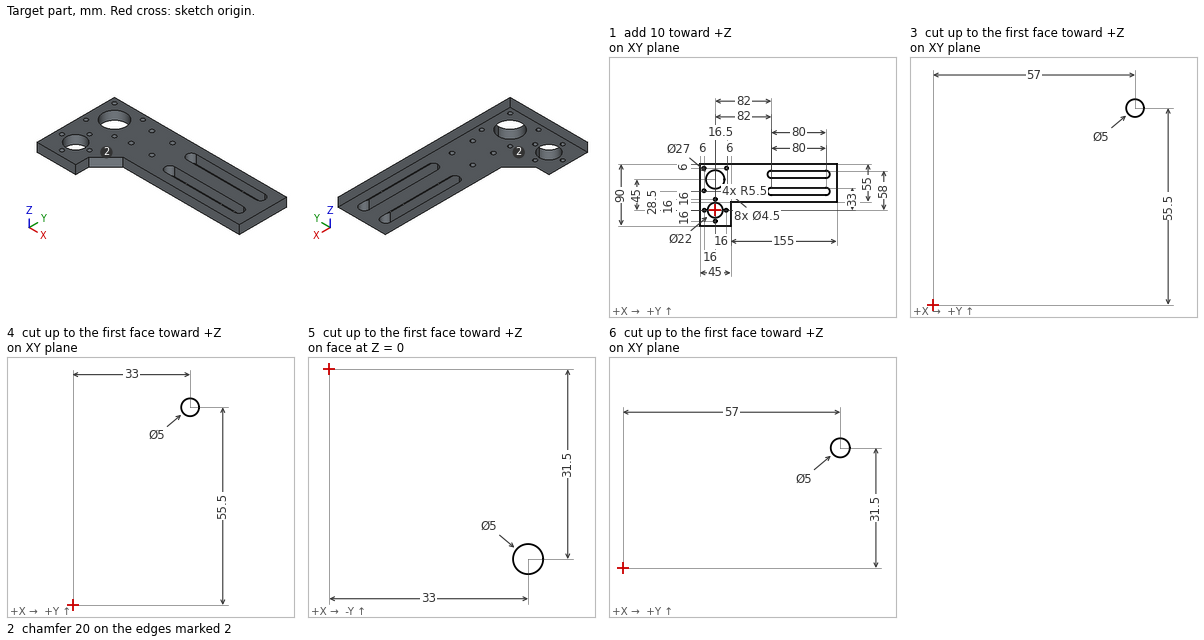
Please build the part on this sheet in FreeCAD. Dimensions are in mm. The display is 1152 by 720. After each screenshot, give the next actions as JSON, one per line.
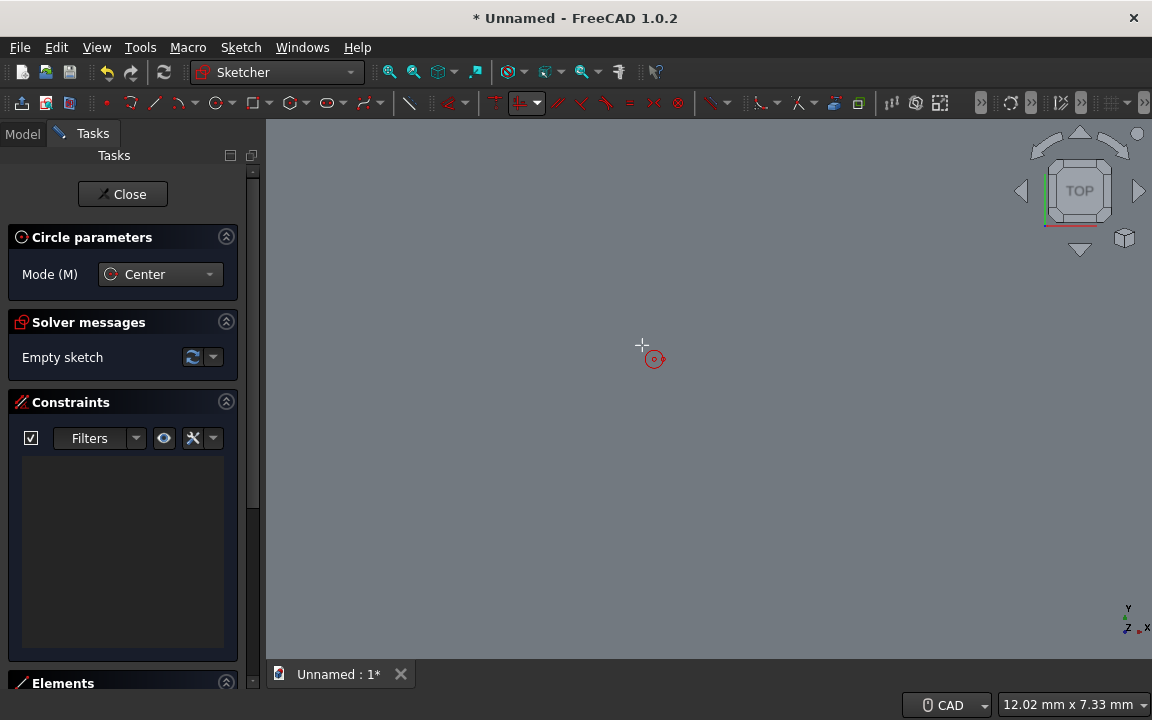
{"action": "left_click", "coordinate": [640, 389]}
{"action": "mouse_move", "coordinate": [771, 258]}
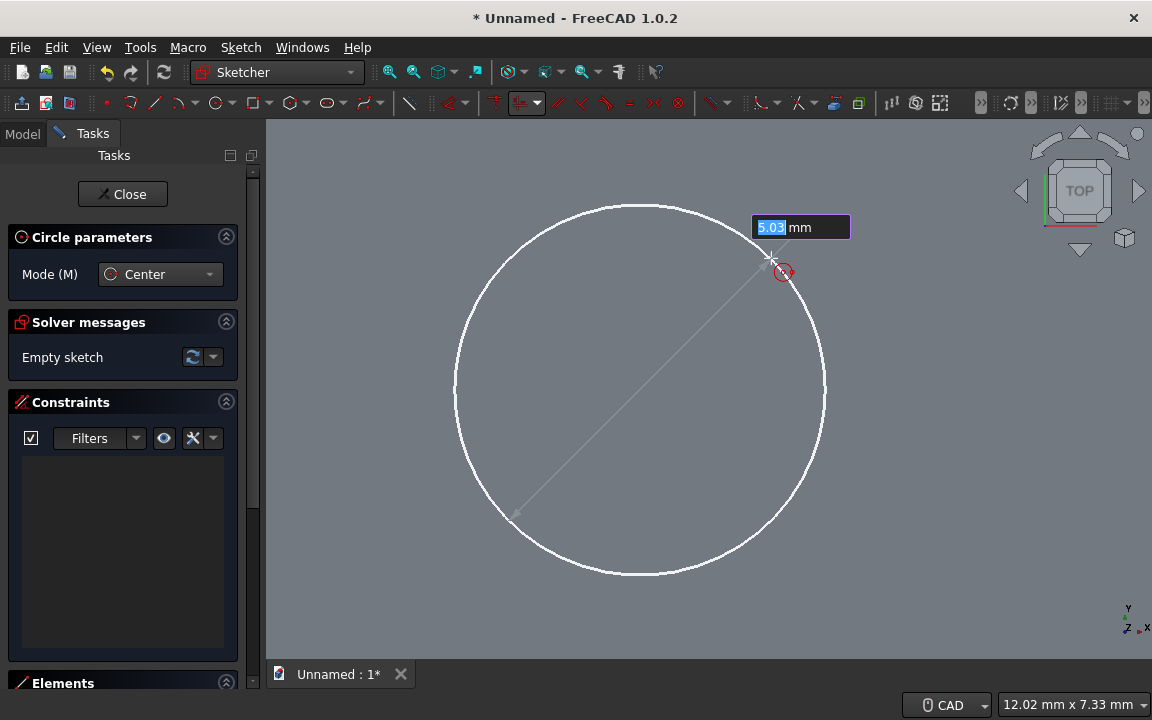
{"action": "type", "text": "5"}
{"action": "key", "text": "Return"}
{"action": "key", "text": "Escape"}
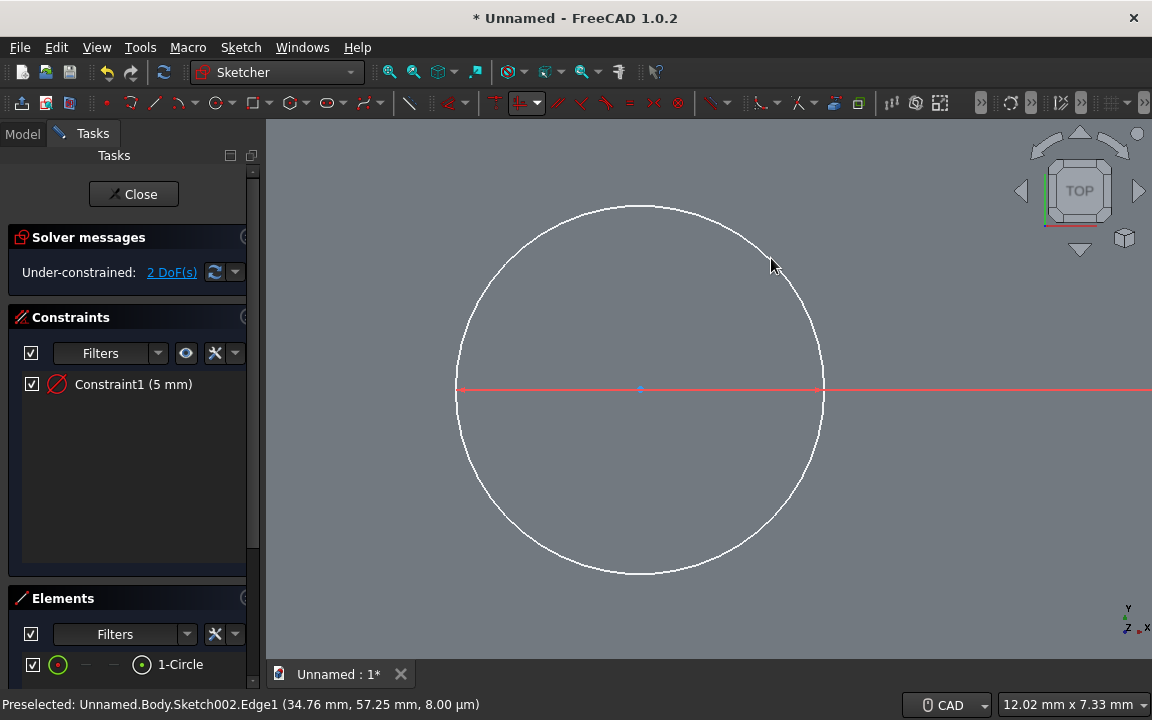
{"action": "key", "text": "d"}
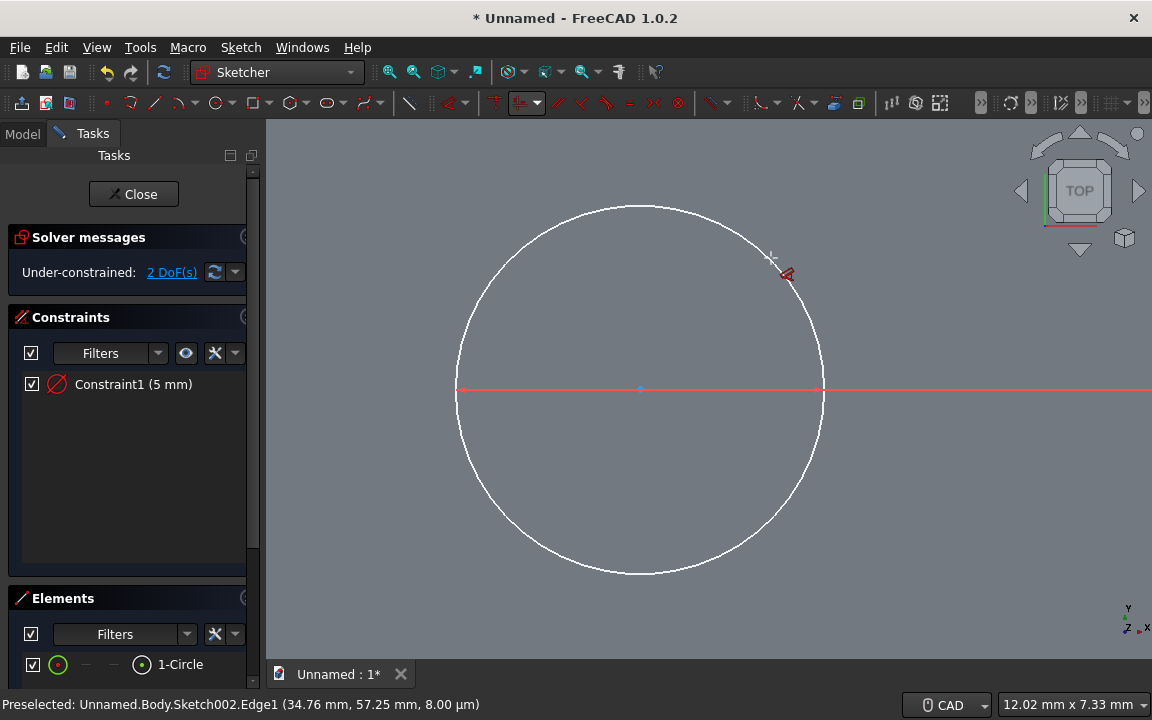
{"action": "left_click", "coordinate": [640, 390]}
{"action": "left_click", "coordinate": [387, 356]}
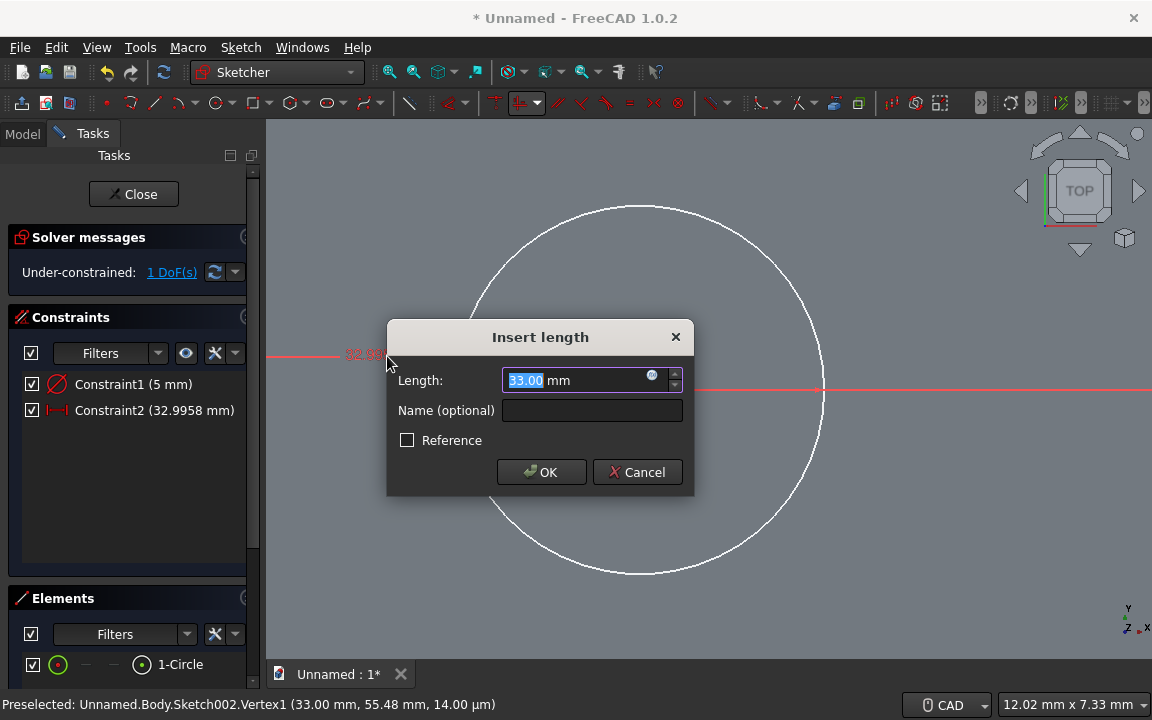
{"action": "type", "text": "33"}
{"action": "key", "text": "Return"}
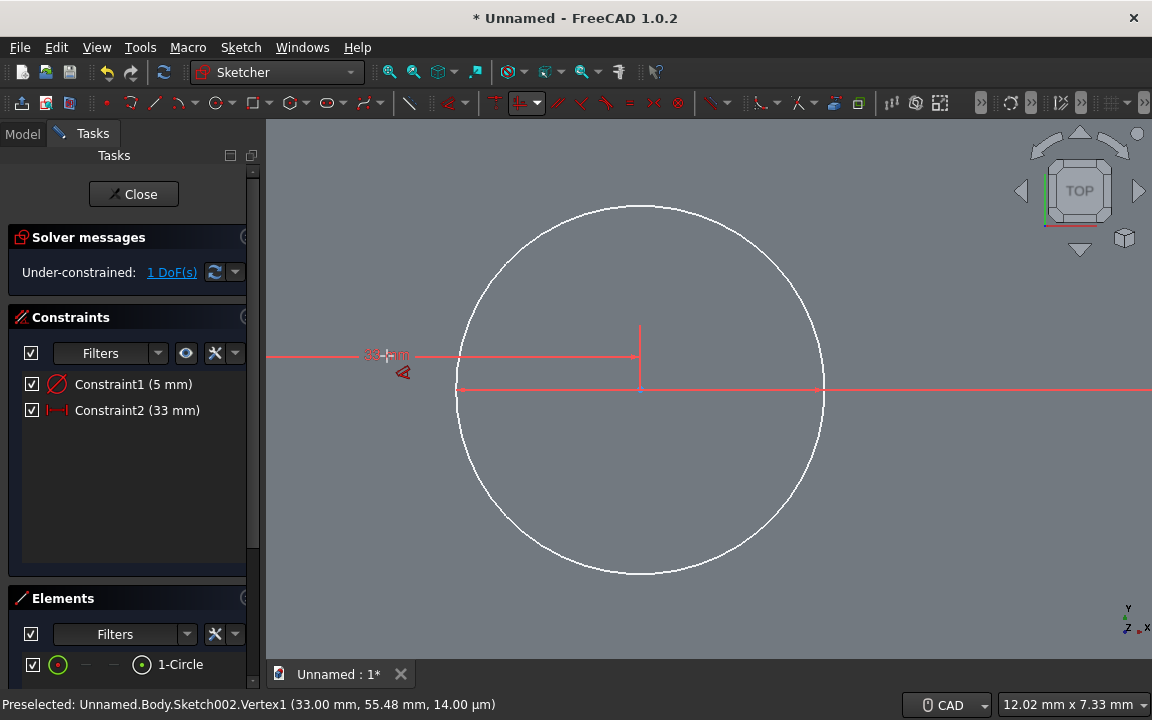
{"action": "left_click", "coordinate": [640, 390]}
{"action": "left_click", "coordinate": [674, 511]}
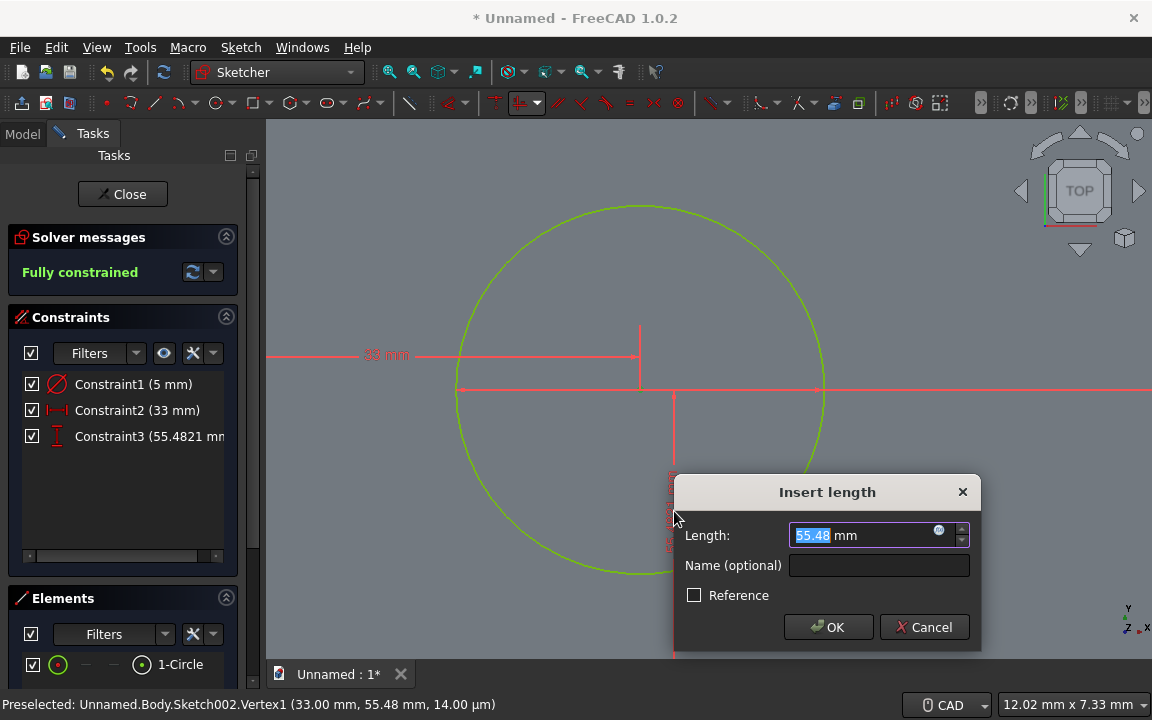
{"action": "type", "text": "55.5"}
{"action": "key", "text": "Return"}
{"action": "key", "text": "Escape"}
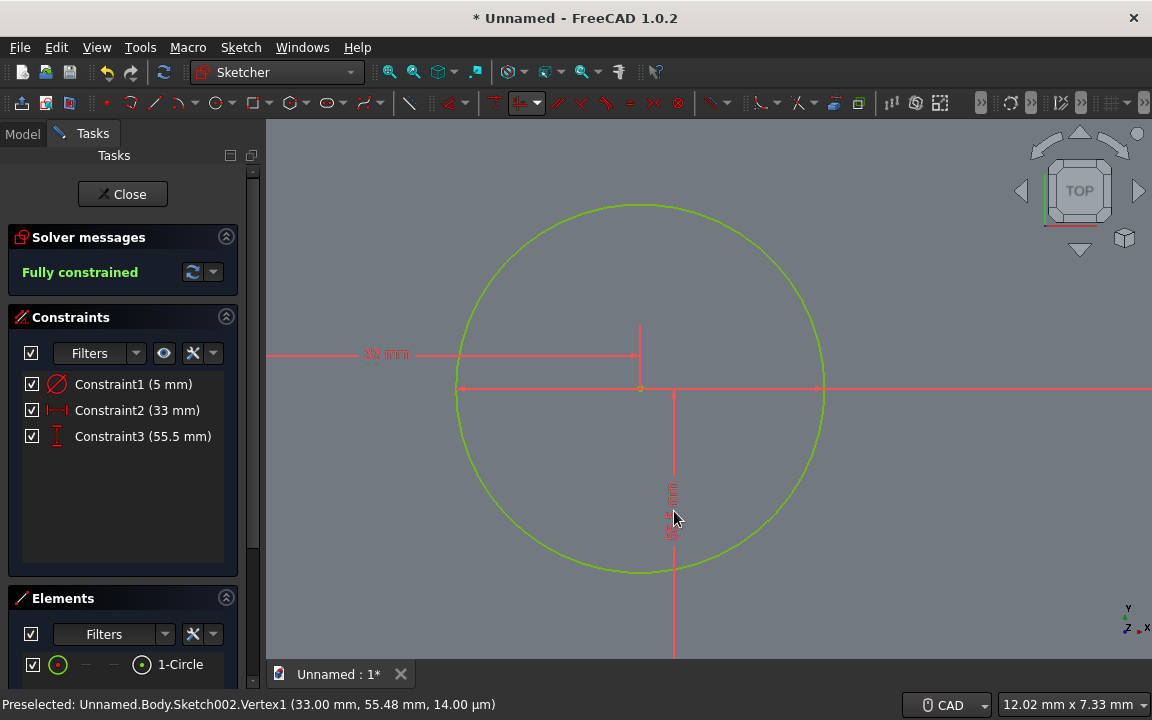
{"action": "left_click", "coordinate": [123, 194]}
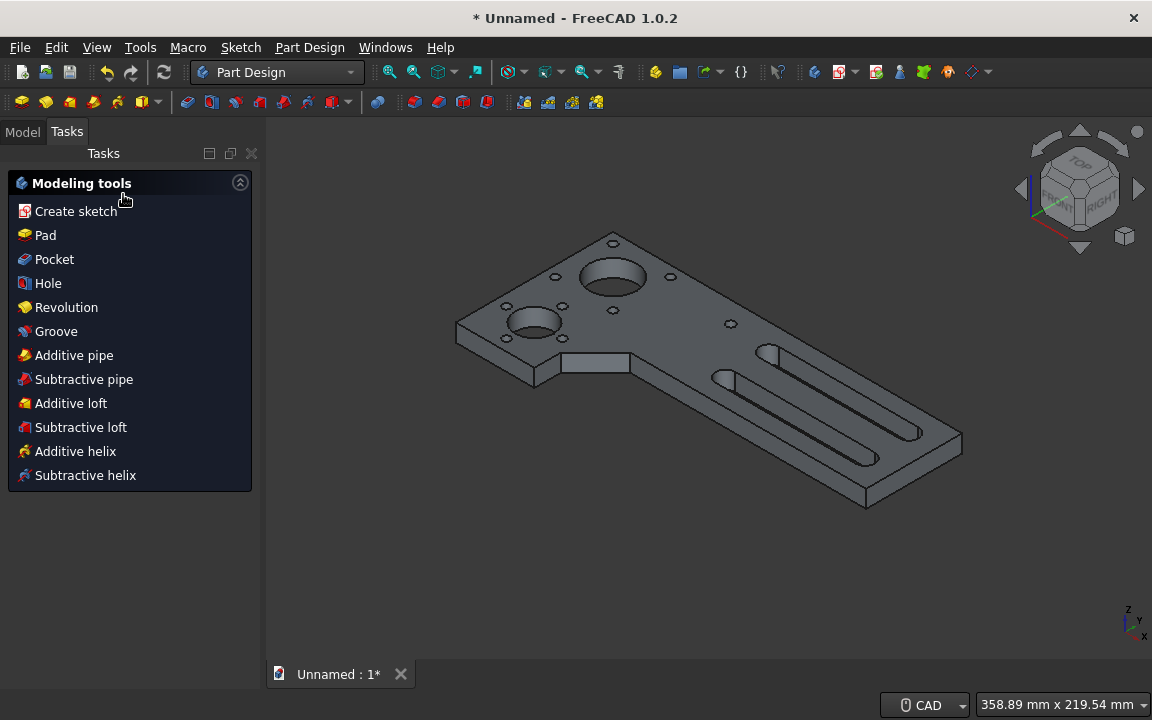
{"action": "left_click", "coordinate": [188, 102]}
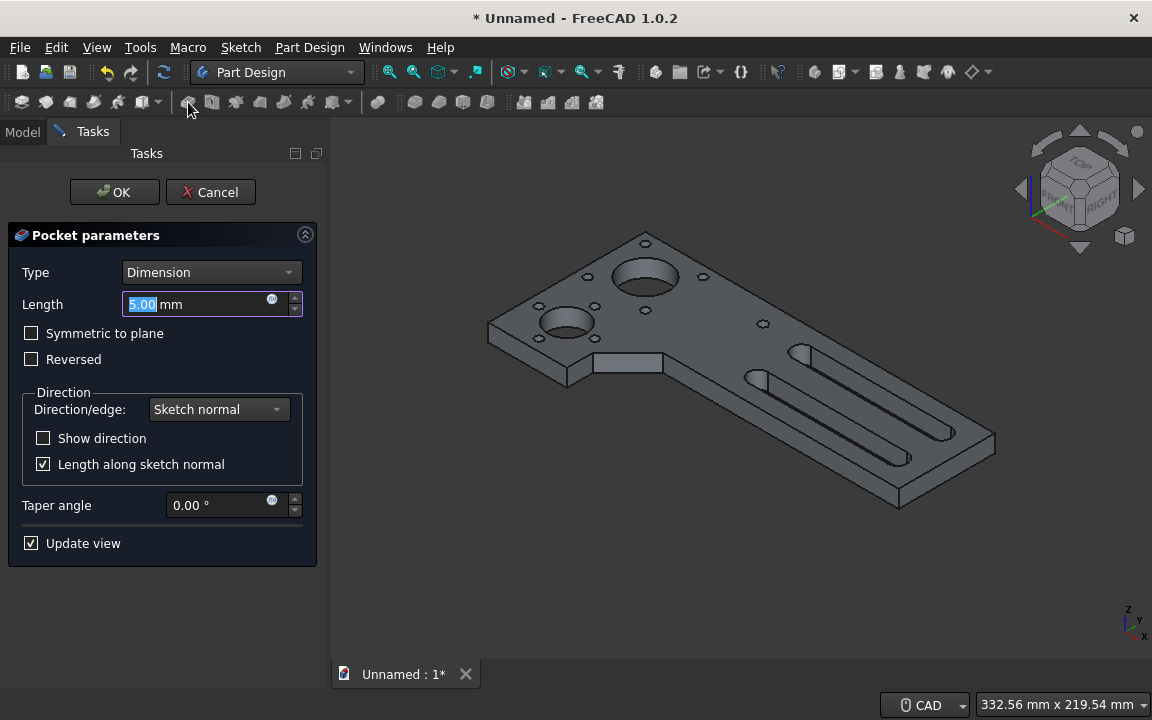
{"action": "left_click", "coordinate": [212, 272]}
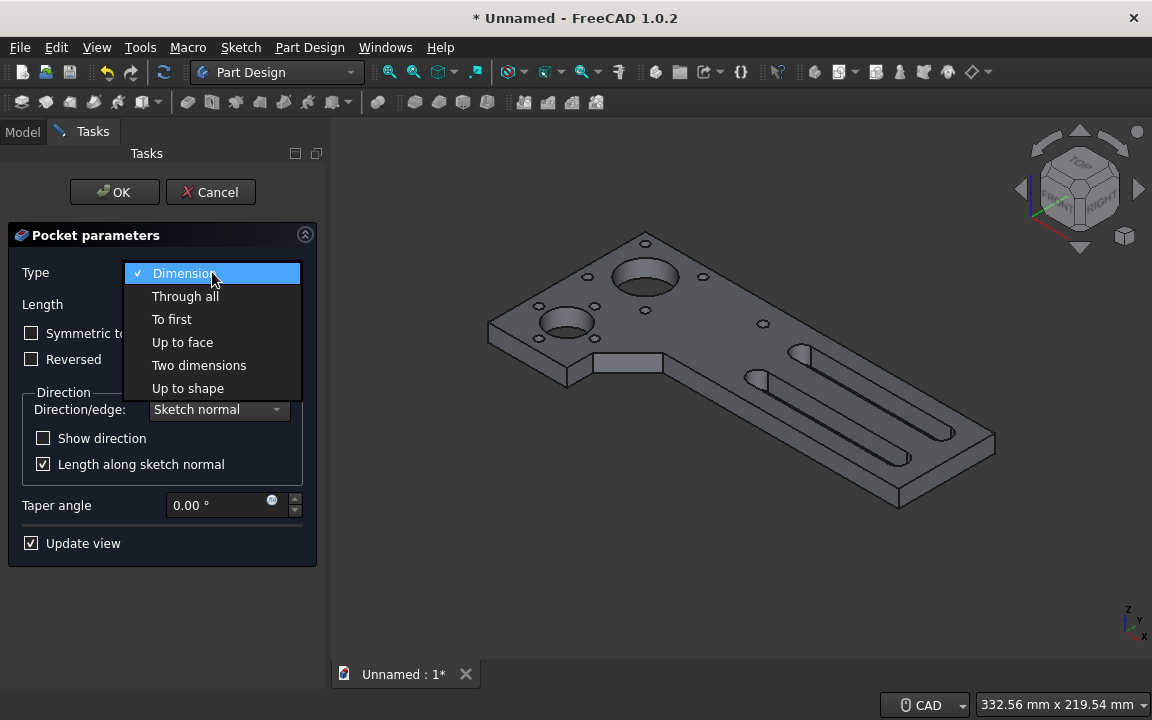
{"action": "left_click", "coordinate": [212, 320]}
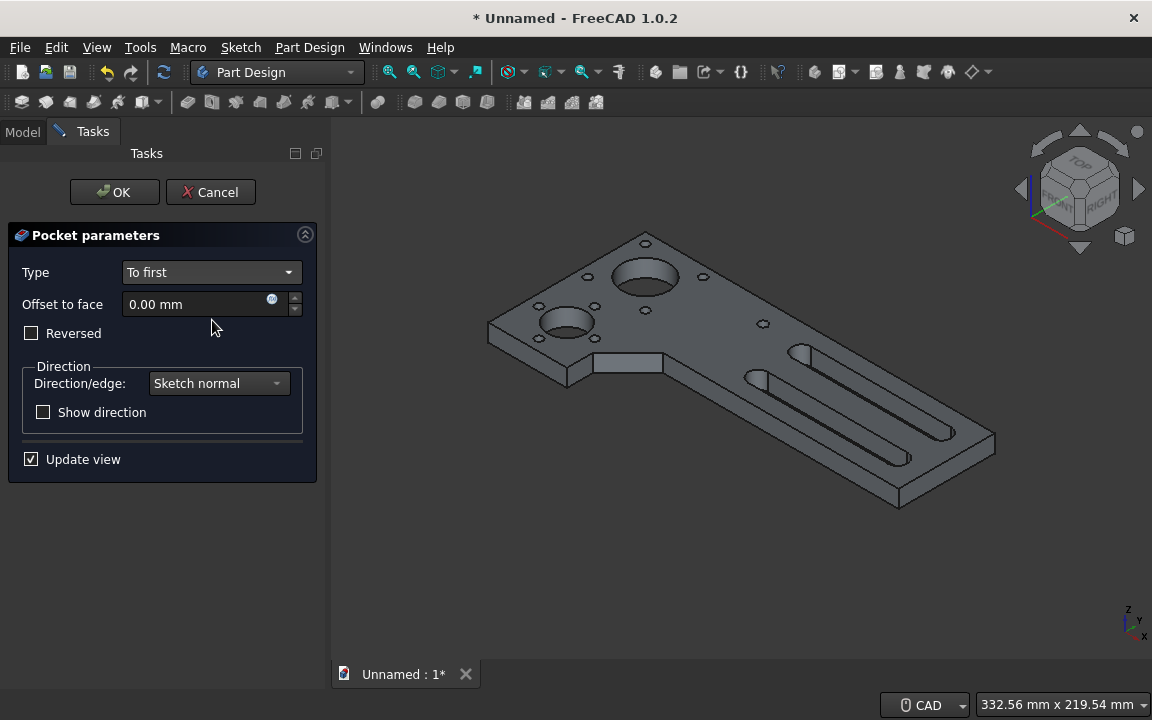
{"action": "left_click", "coordinate": [30, 333]}